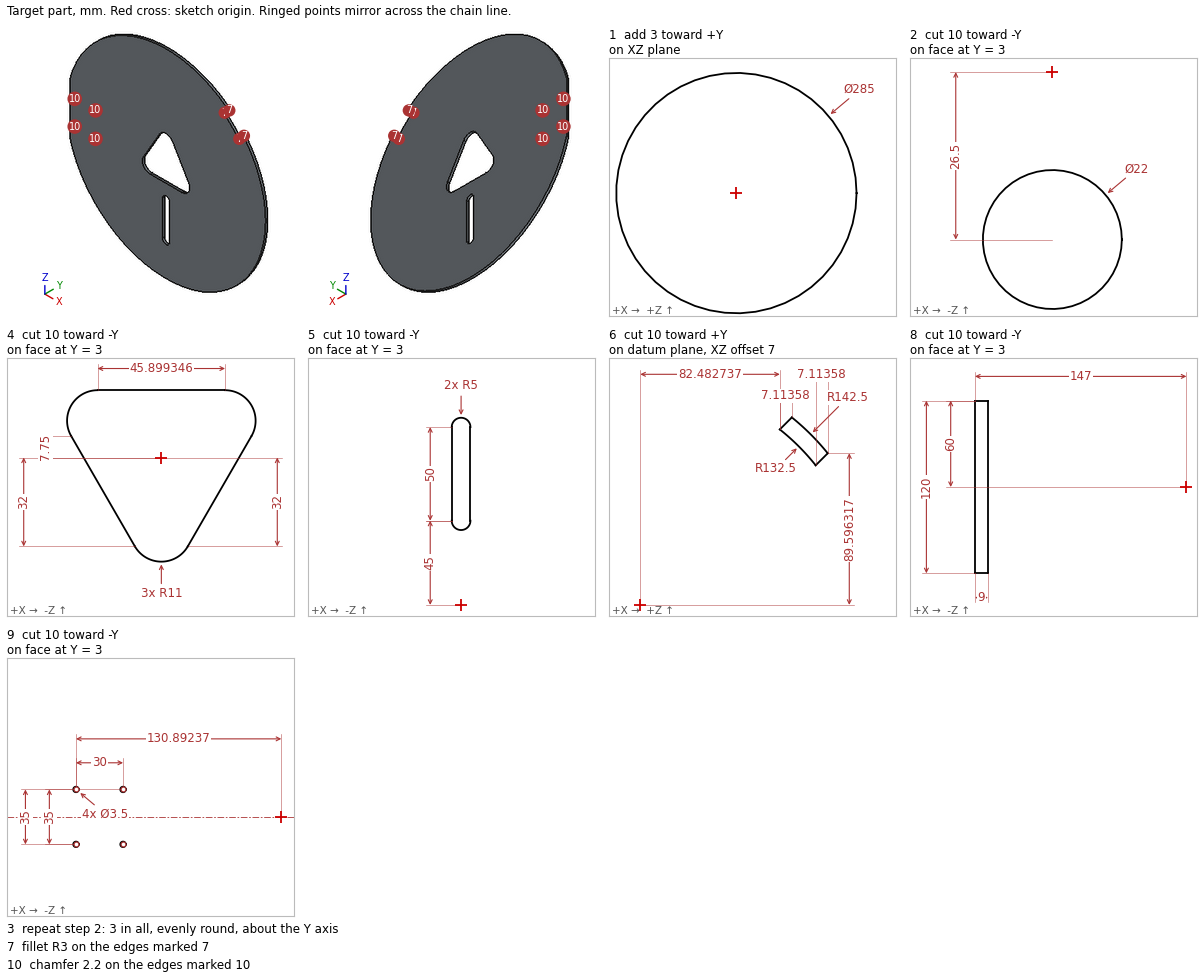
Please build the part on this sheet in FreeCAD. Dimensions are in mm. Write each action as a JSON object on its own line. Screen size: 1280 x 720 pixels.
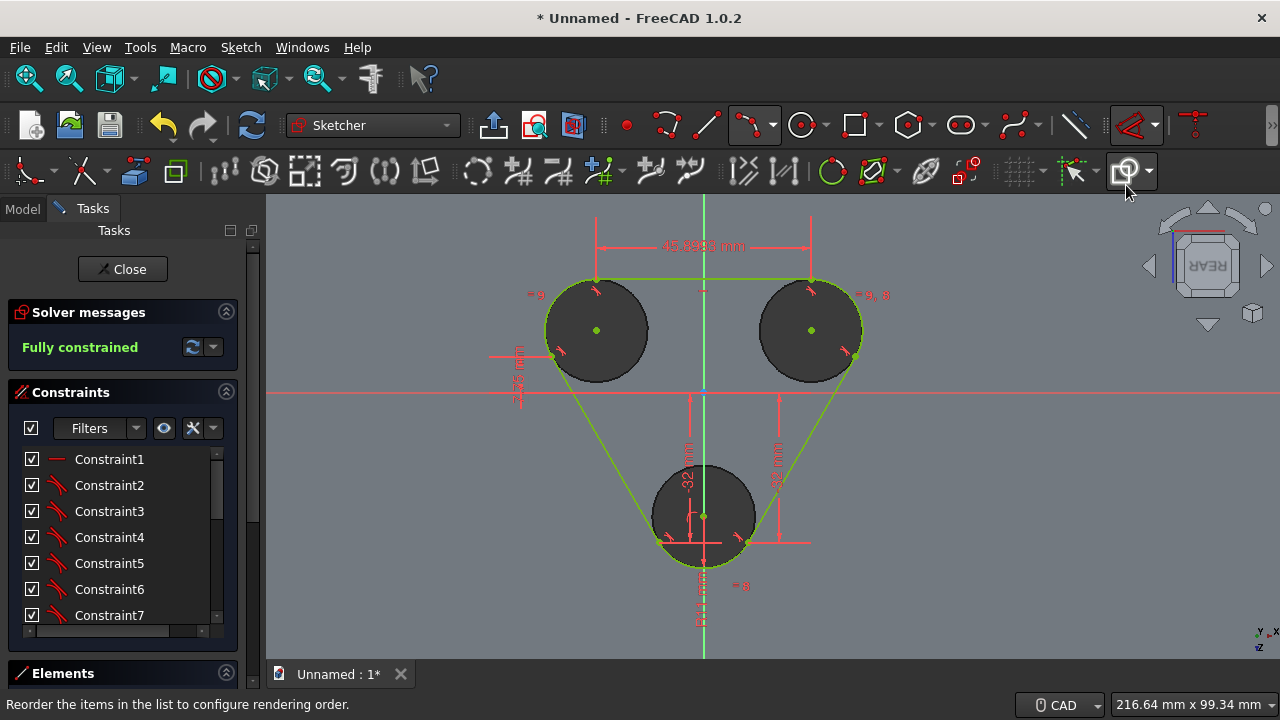
{"action": "left_click", "coordinate": [123, 269]}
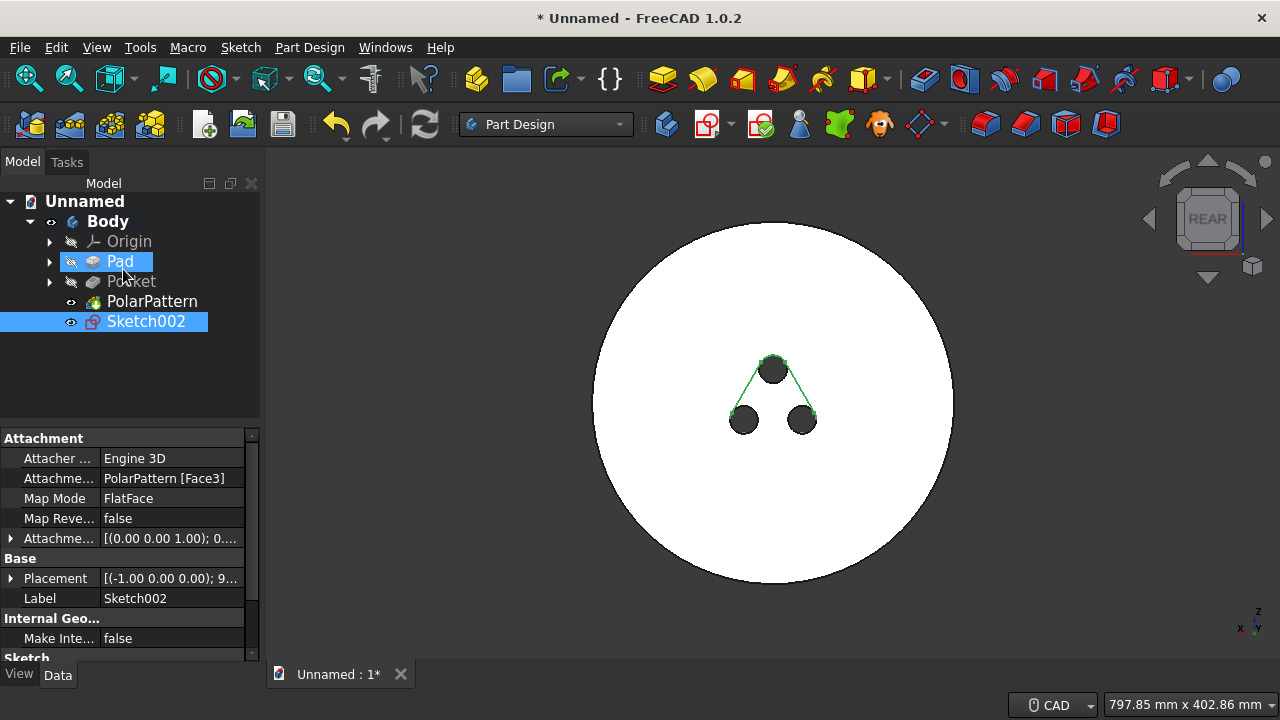
{"action": "left_click", "coordinate": [926, 80]}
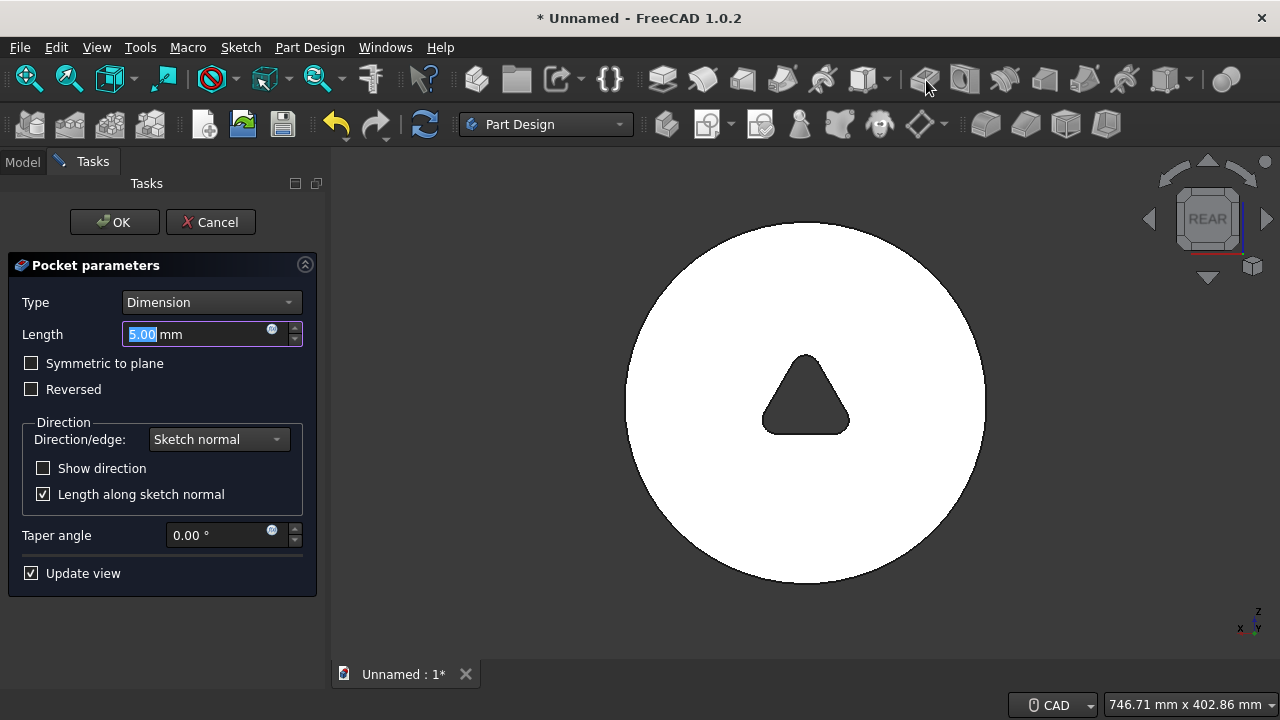
{"action": "type", "text": "10"}
{"action": "key", "text": "Tab"}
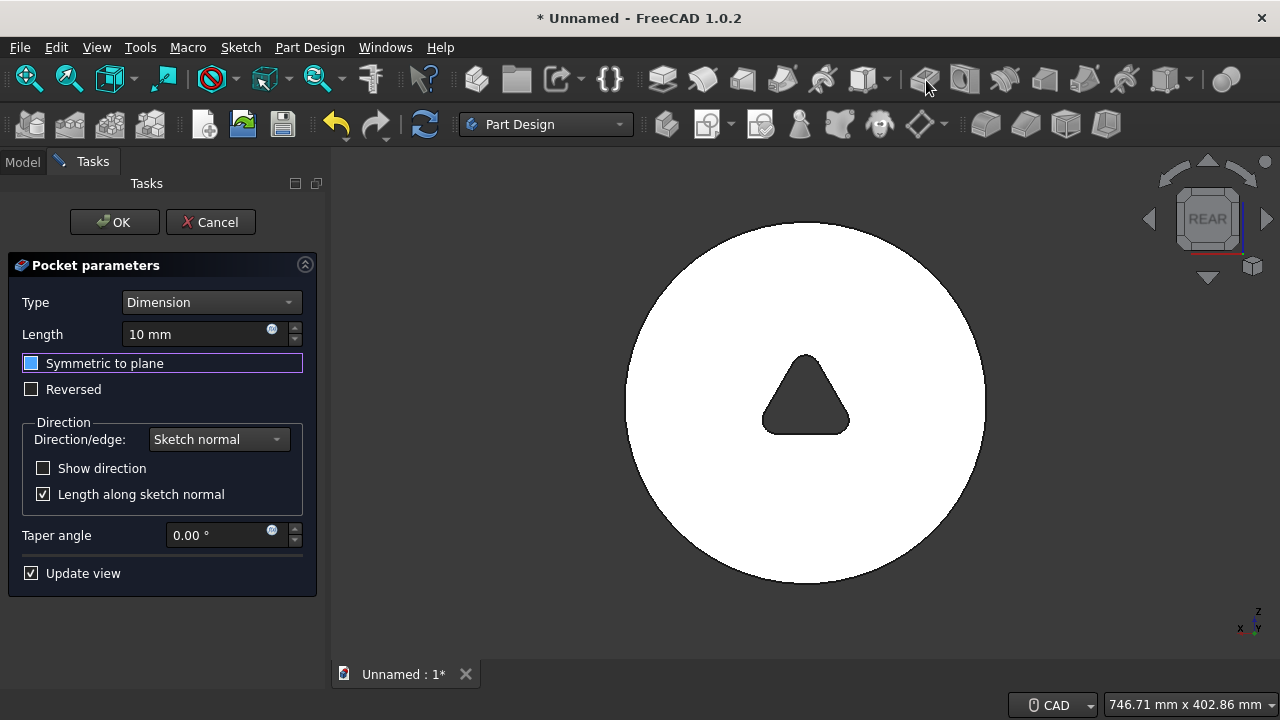
{"action": "left_click", "coordinate": [115, 222]}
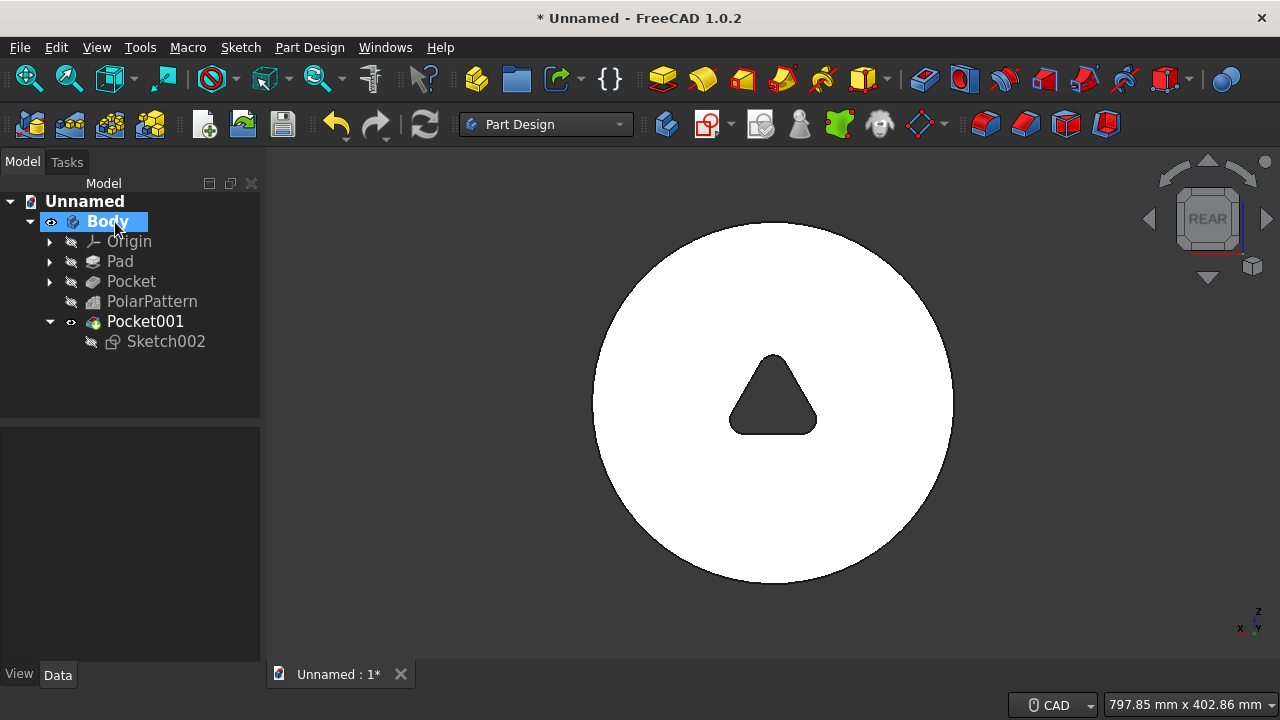
{"action": "left_click", "coordinate": [773, 505]}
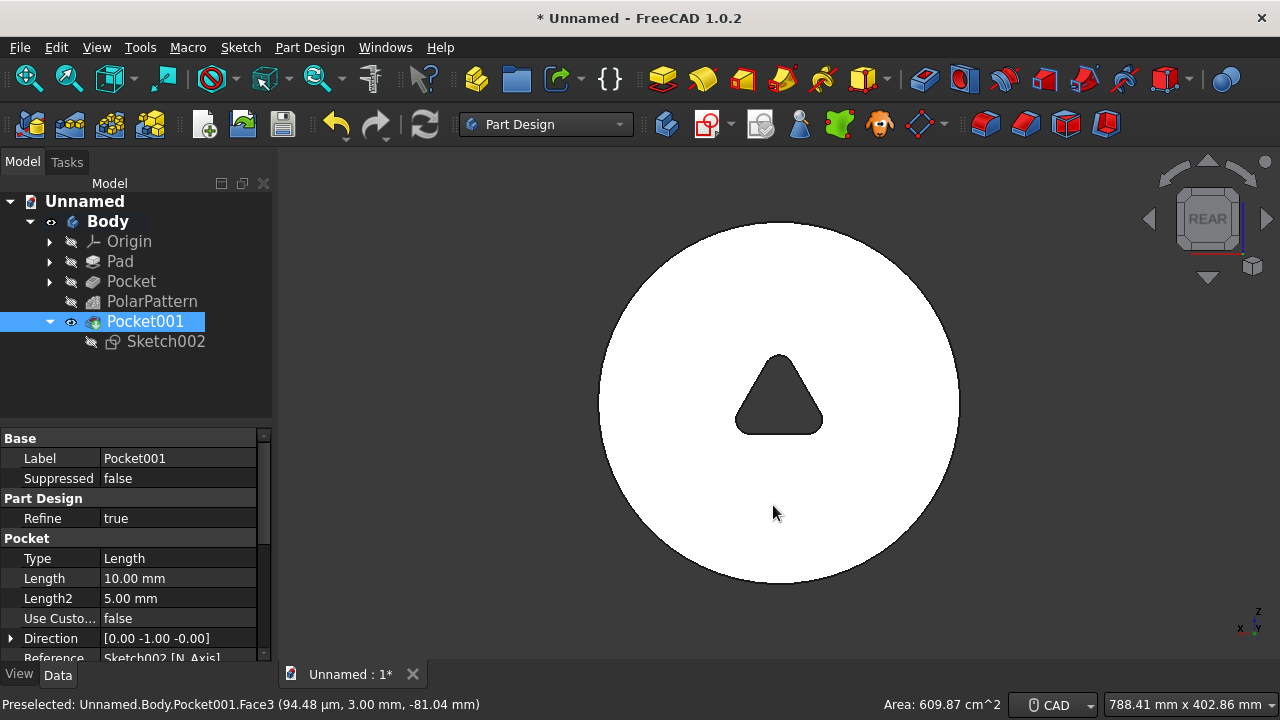
{"action": "left_click", "coordinate": [708, 124]}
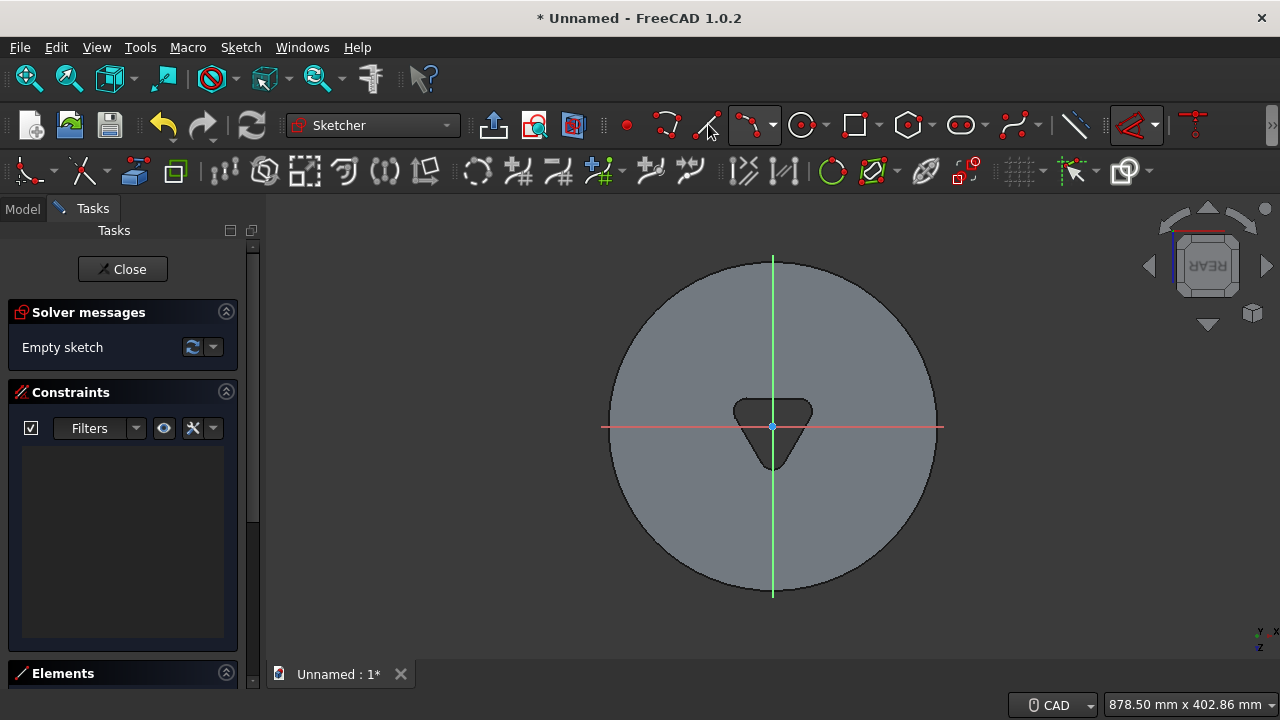
{"action": "scroll", "coordinate": [813, 335], "scroll_direction": "up", "scroll_amount": 5}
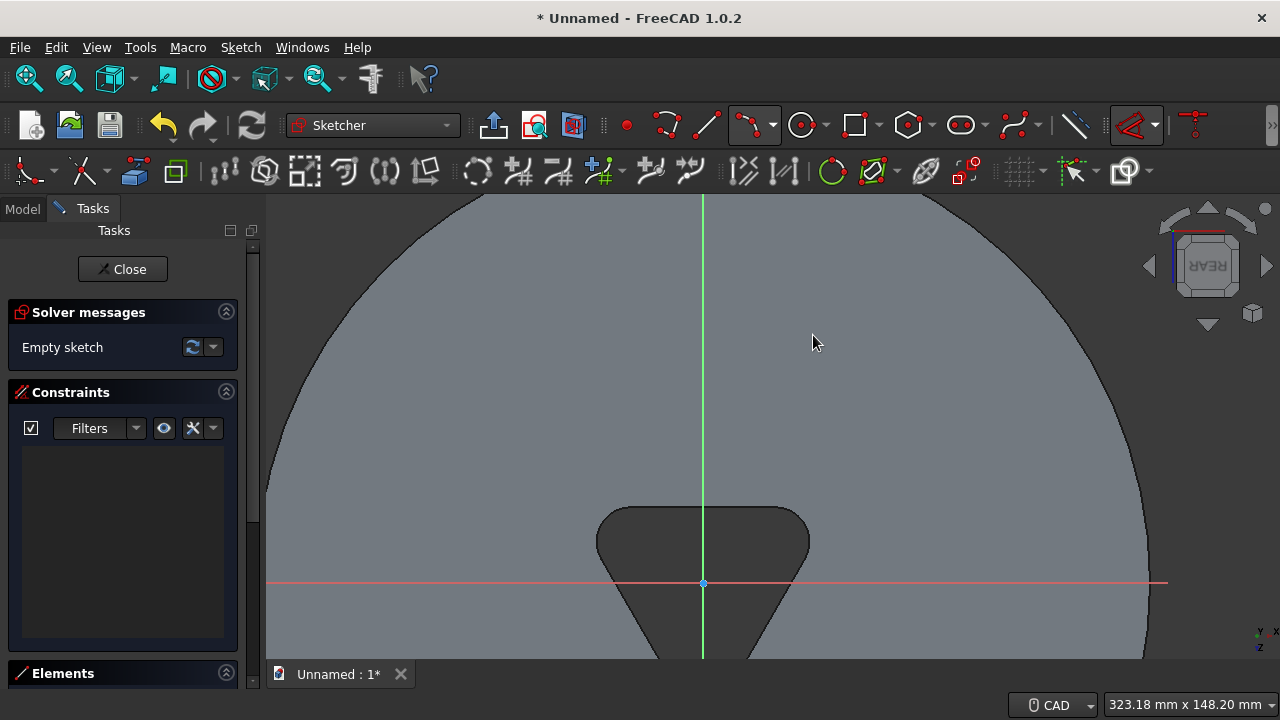
{"action": "left_click", "coordinate": [962, 126]}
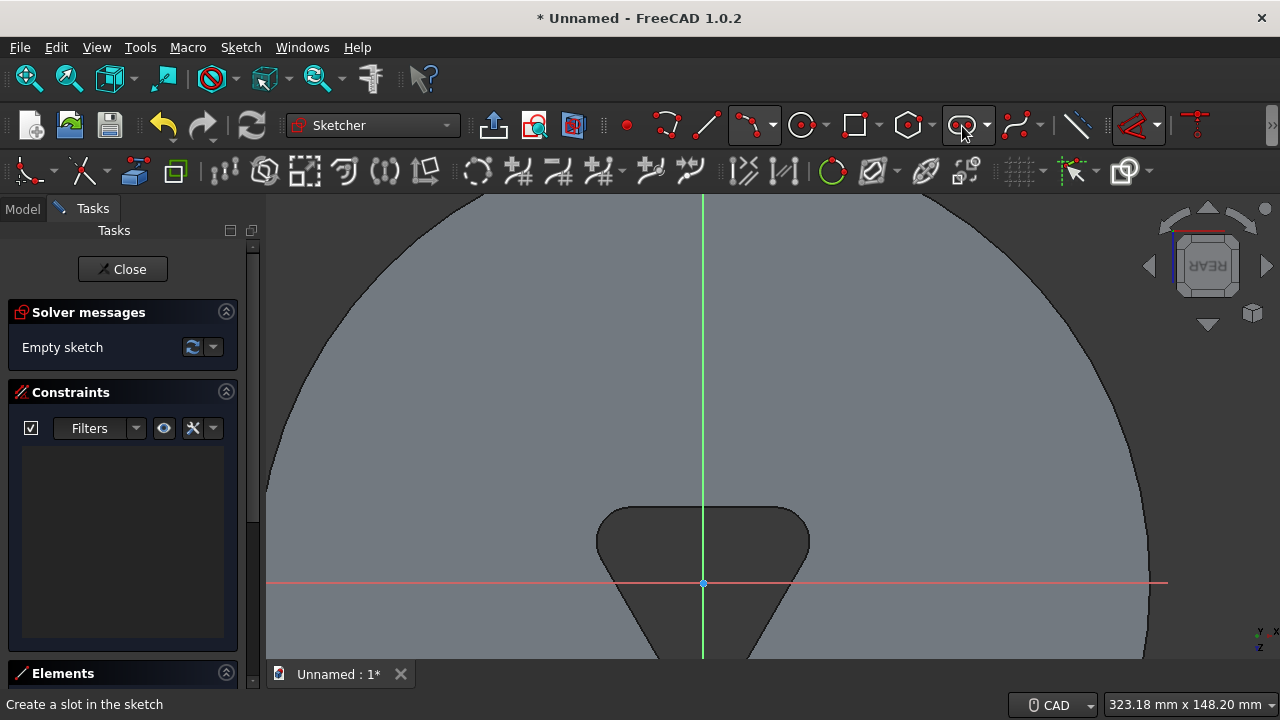
{"action": "scroll", "coordinate": [703, 442], "scroll_direction": "up", "scroll_amount": 2}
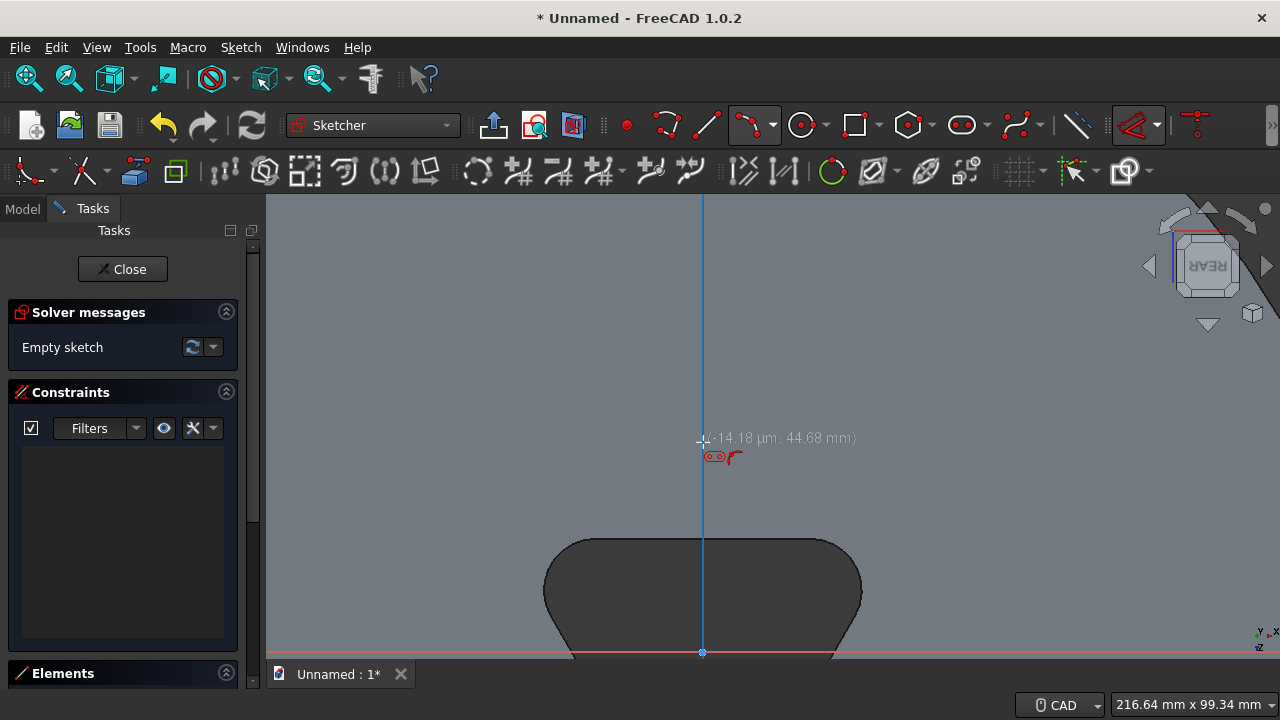
{"action": "left_click", "coordinate": [703, 442]}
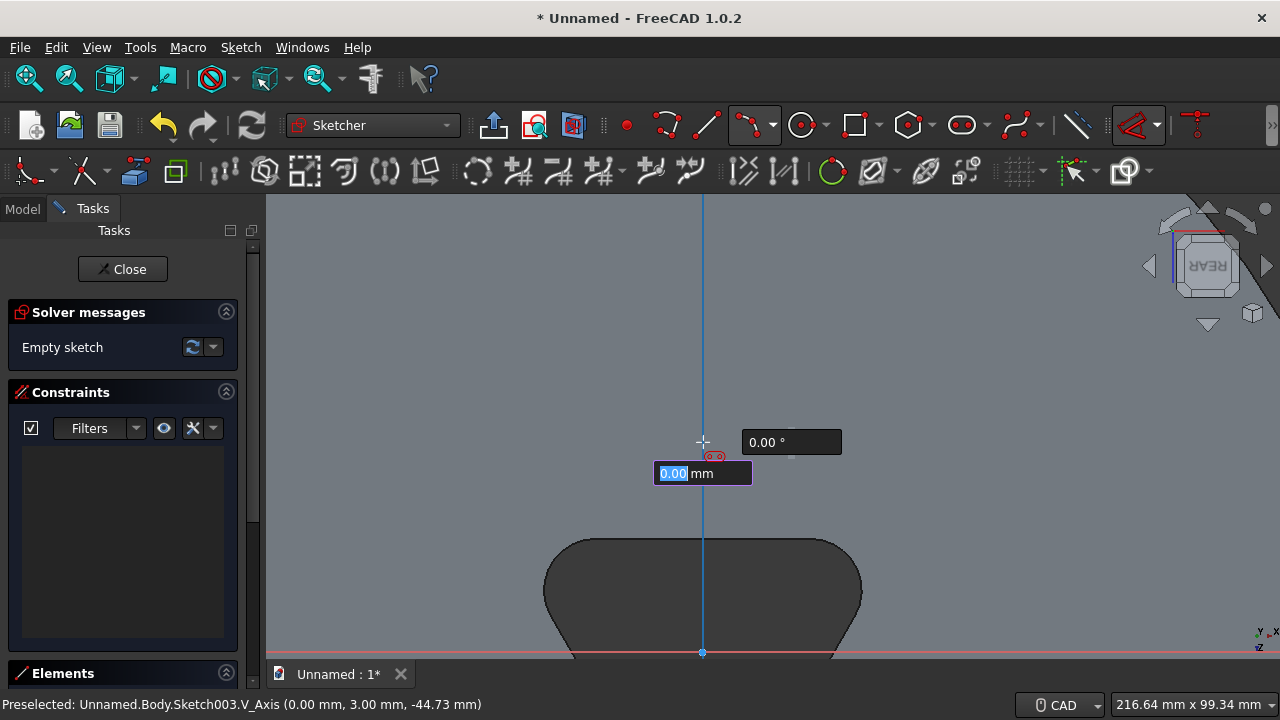
{"action": "scroll", "coordinate": [708, 443], "scroll_direction": "down", "scroll_amount": 2}